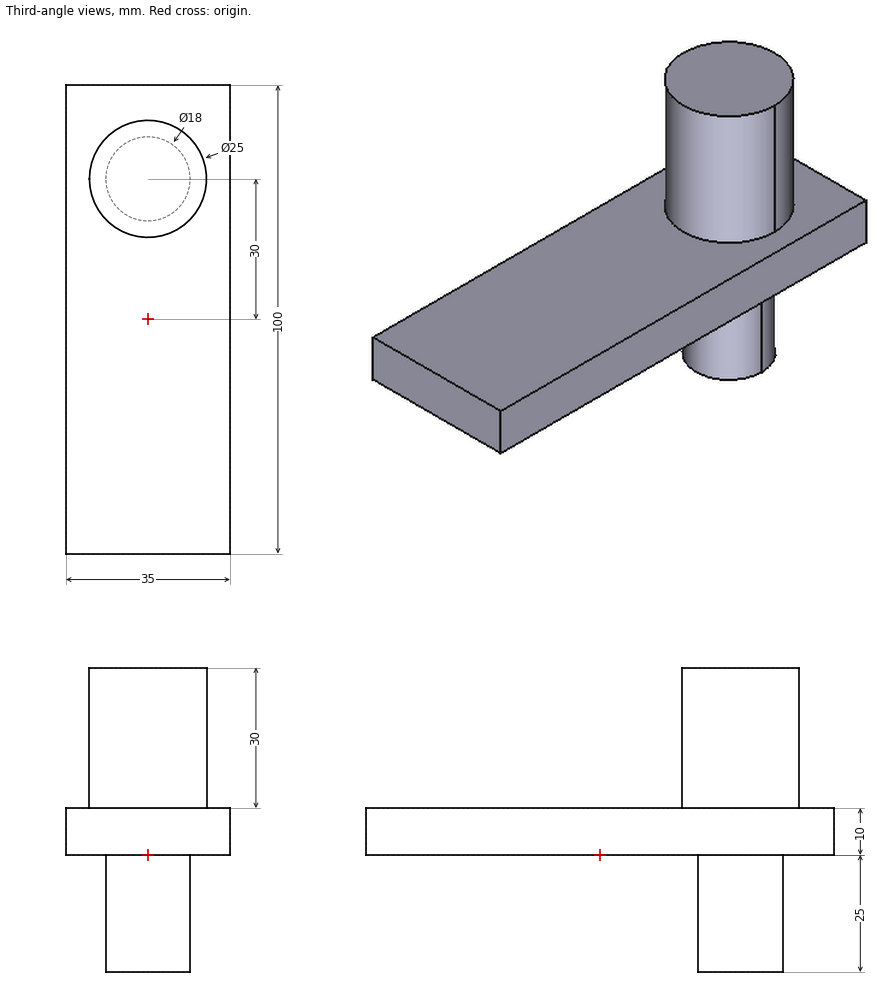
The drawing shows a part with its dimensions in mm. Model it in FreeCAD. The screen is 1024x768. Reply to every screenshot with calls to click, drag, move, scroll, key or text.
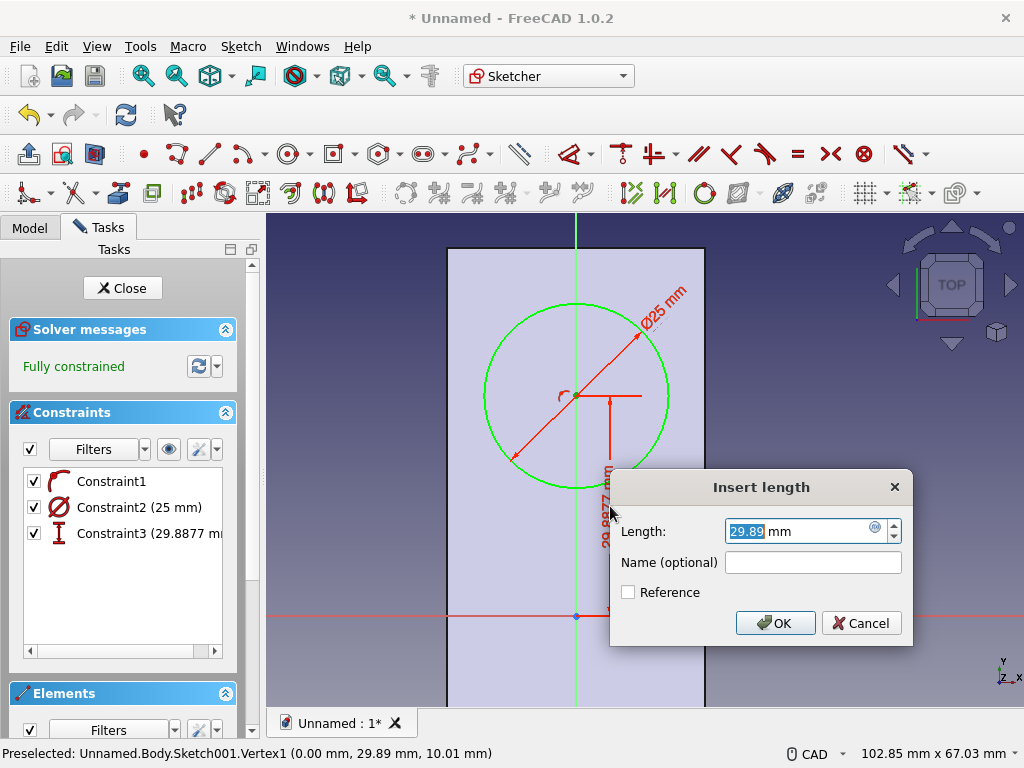
text(30)
key(Return)
key(Escape)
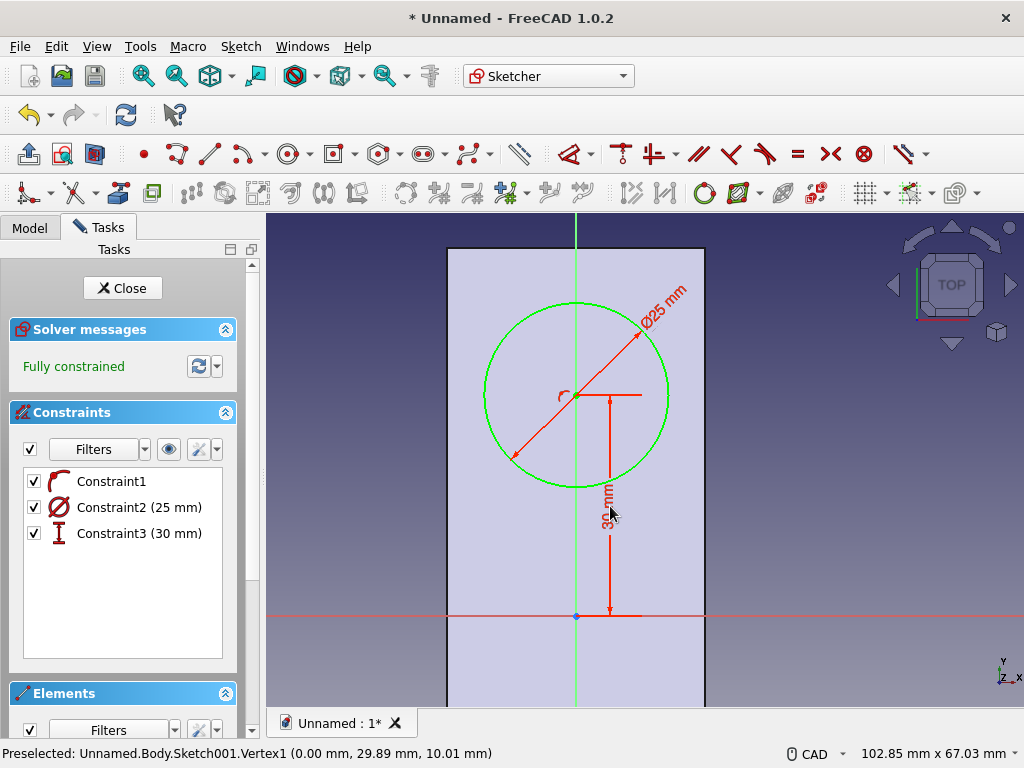
click(123, 288)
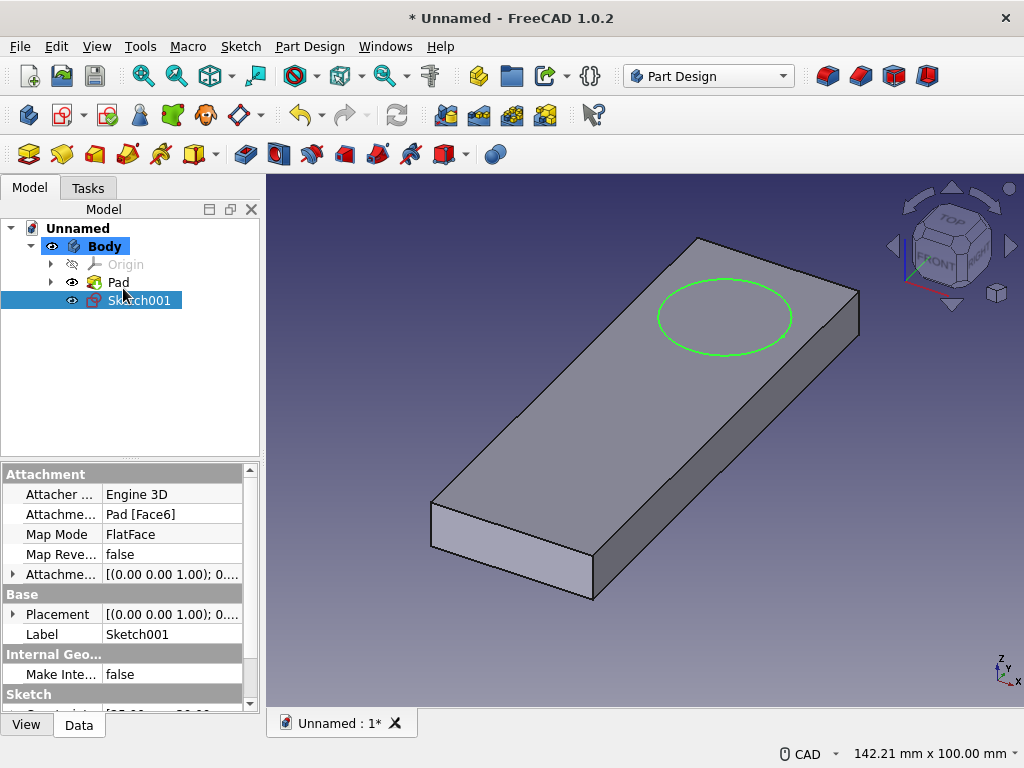
click(29, 154)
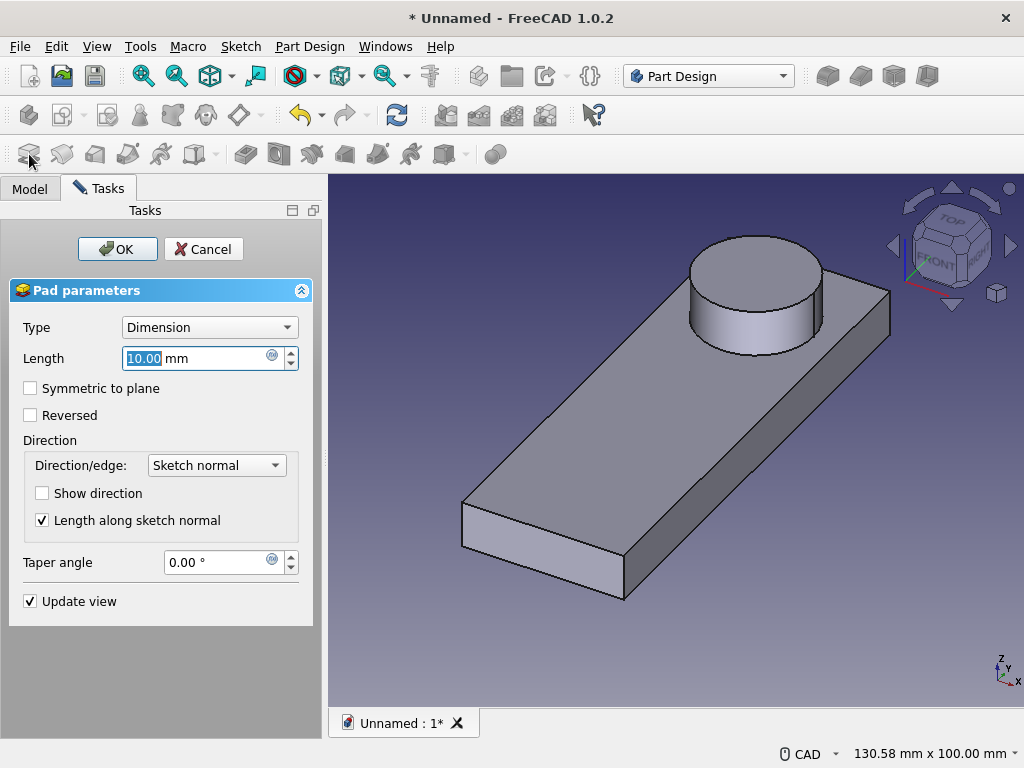
text(30)
key(Tab)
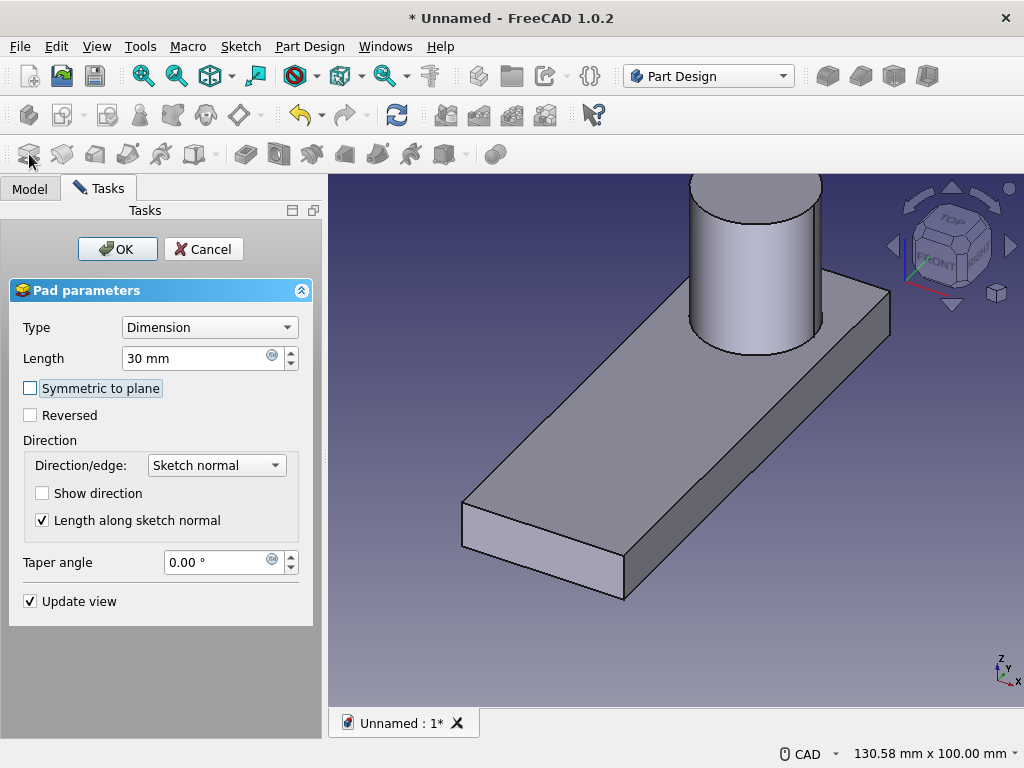
click(118, 249)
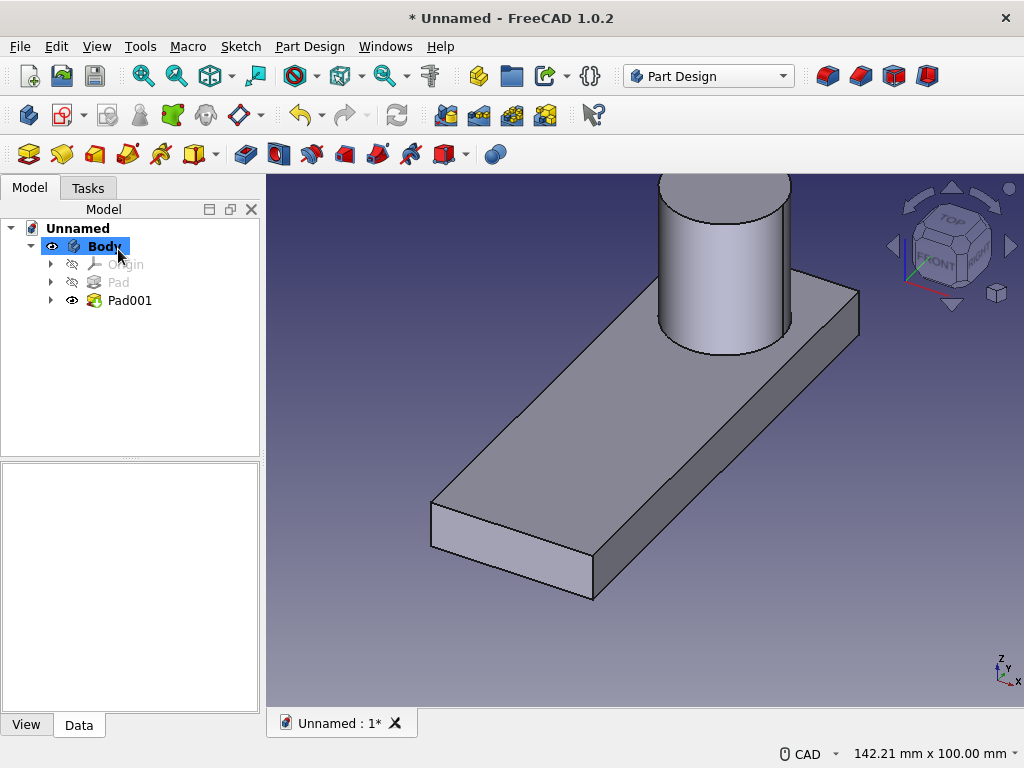
click(144, 76)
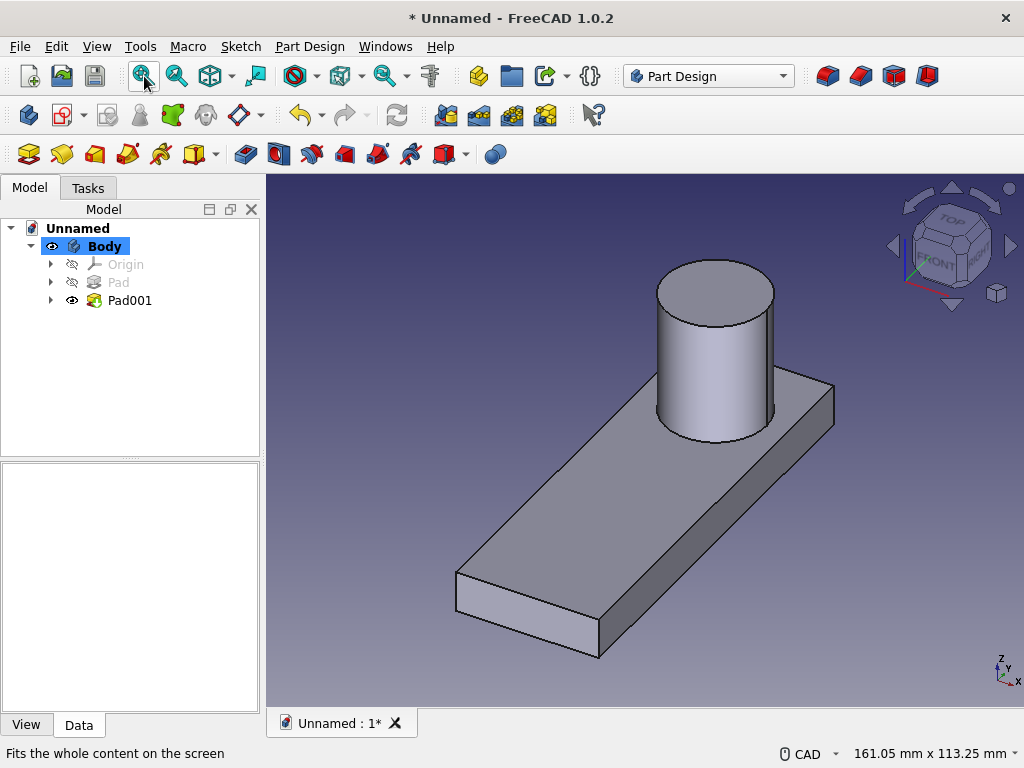
click(62, 116)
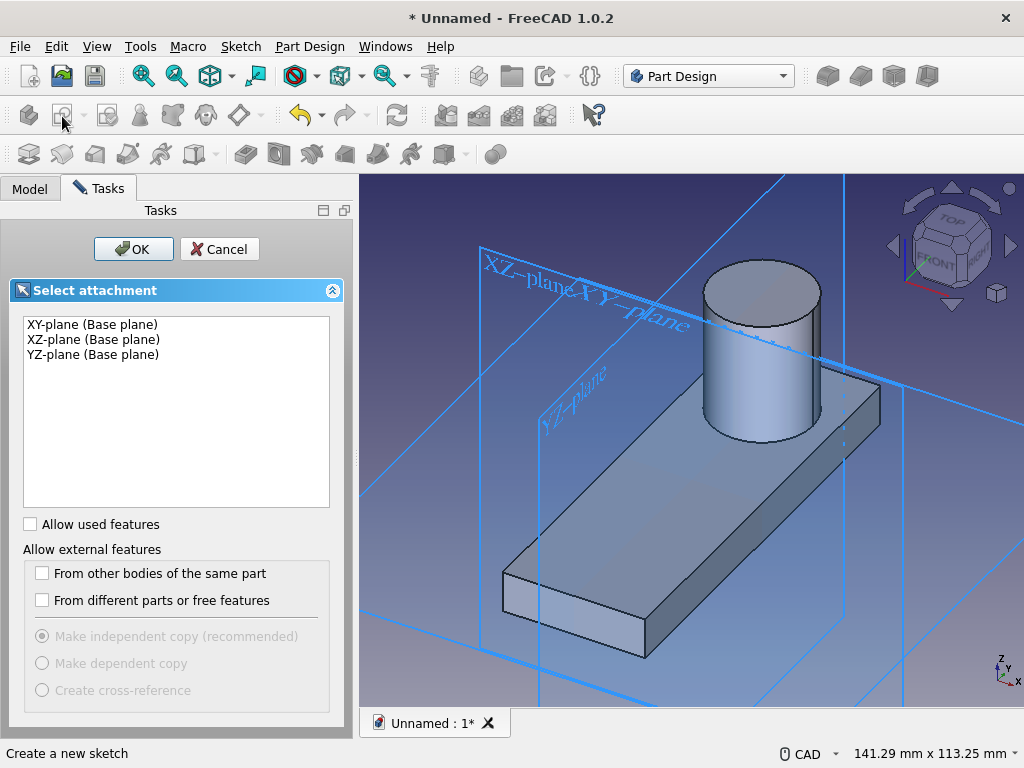
click(84, 324)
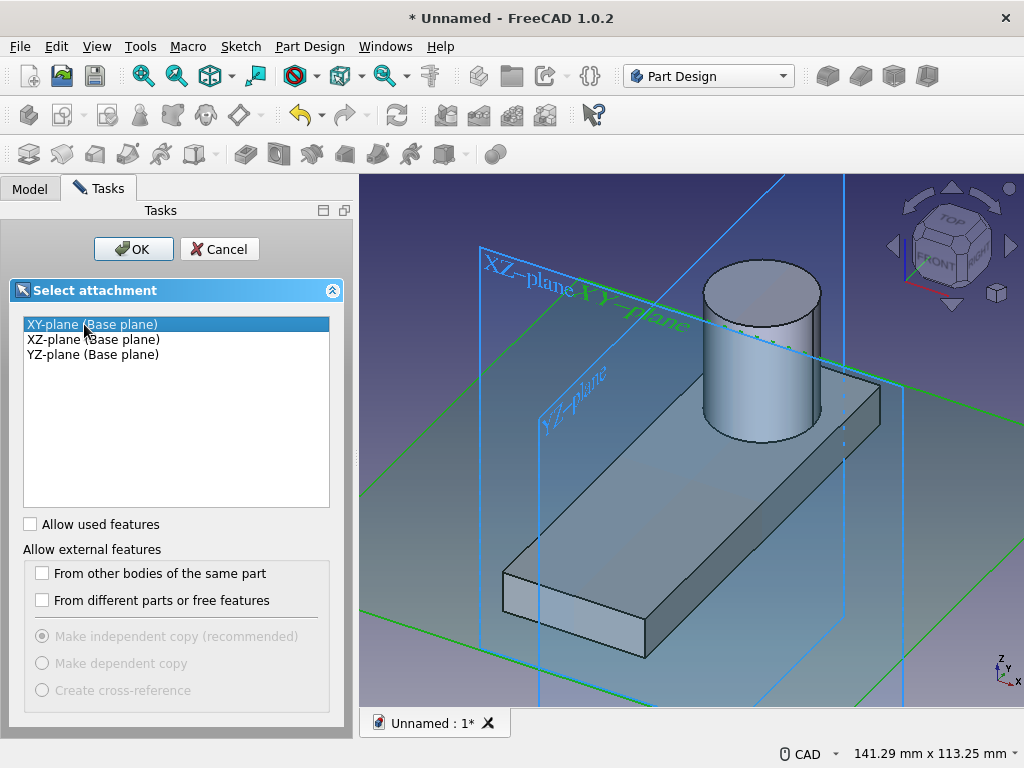
click(134, 249)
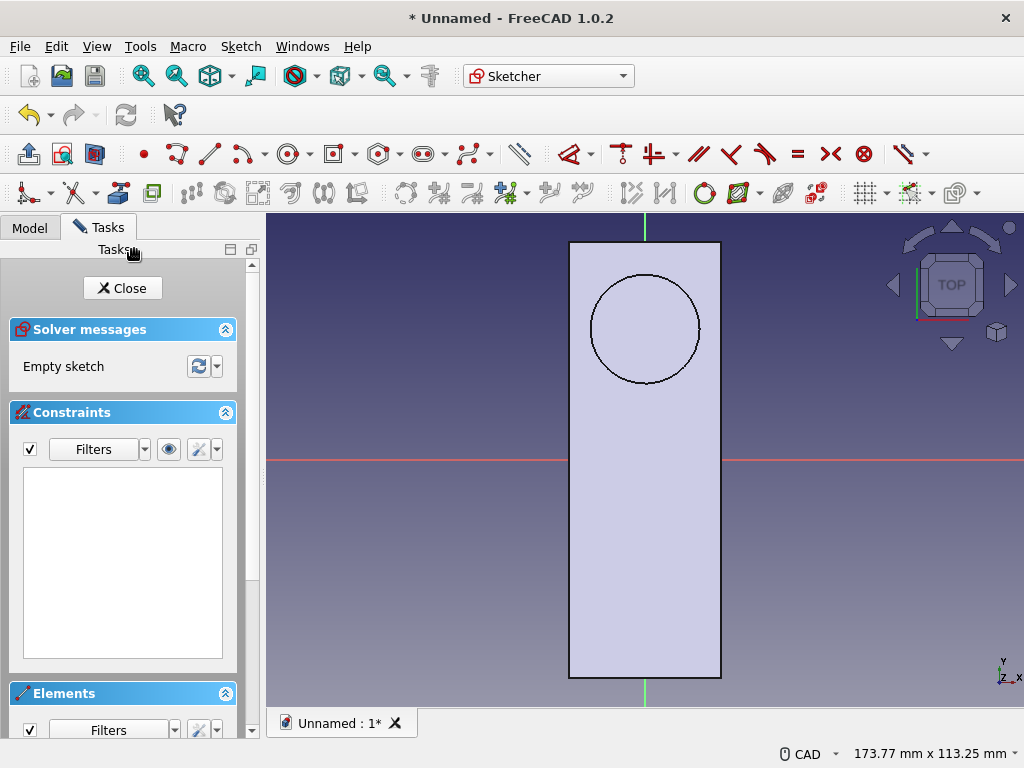
click(95, 154)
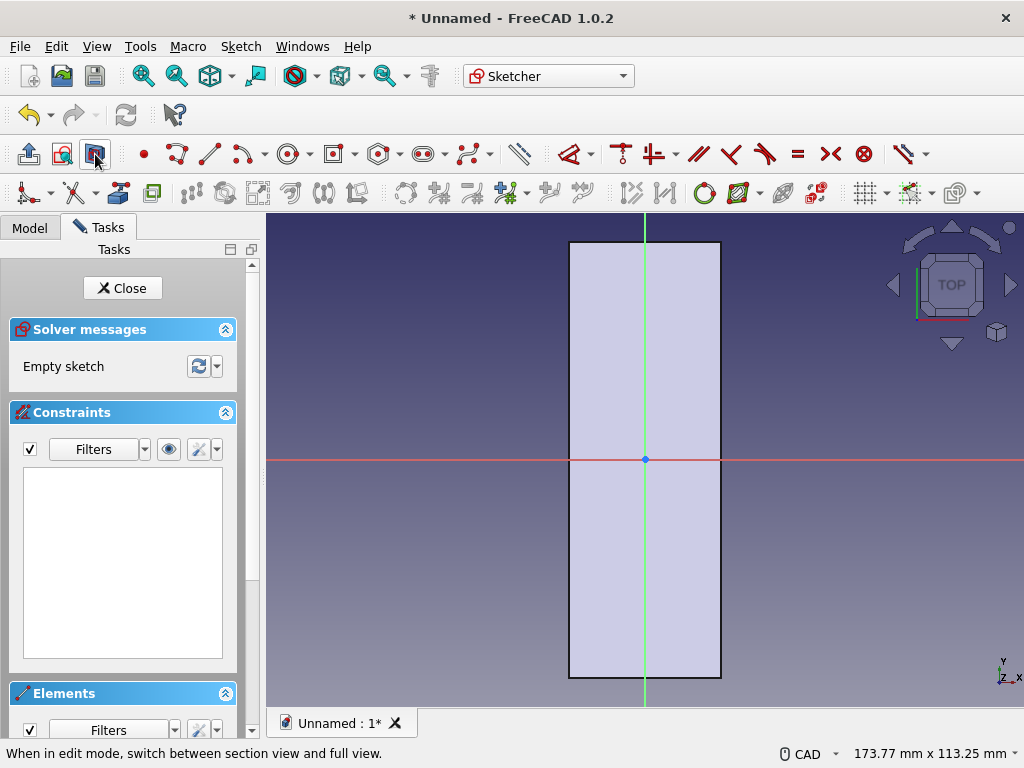
scroll(728, 271, up, 3)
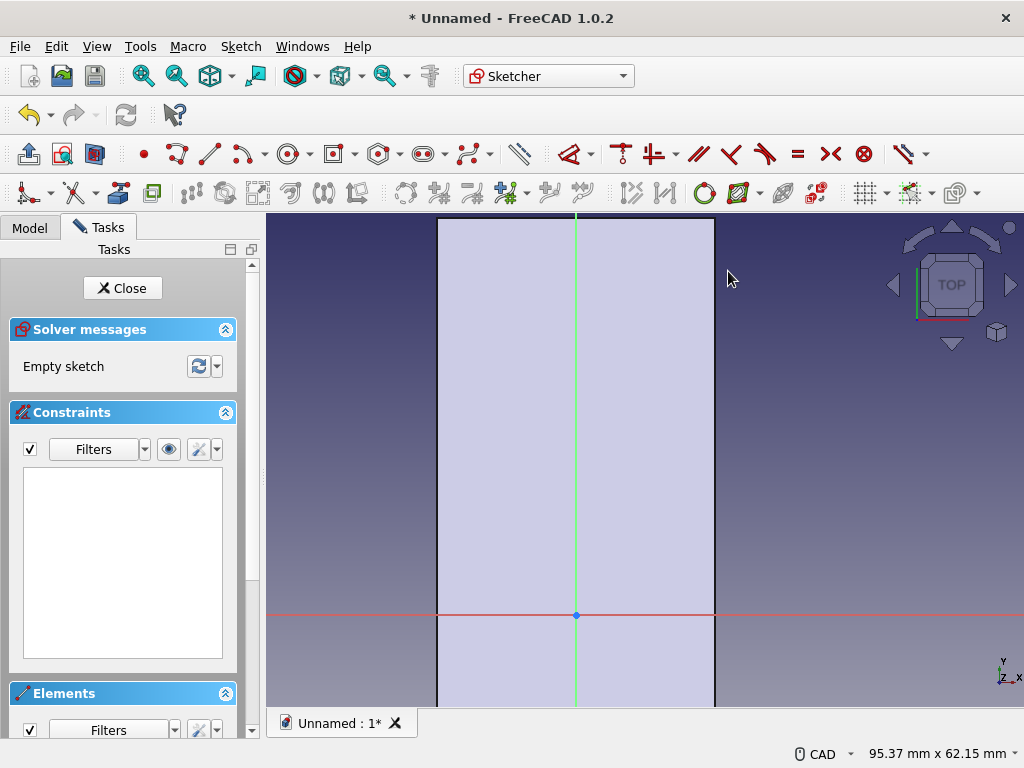
click(288, 154)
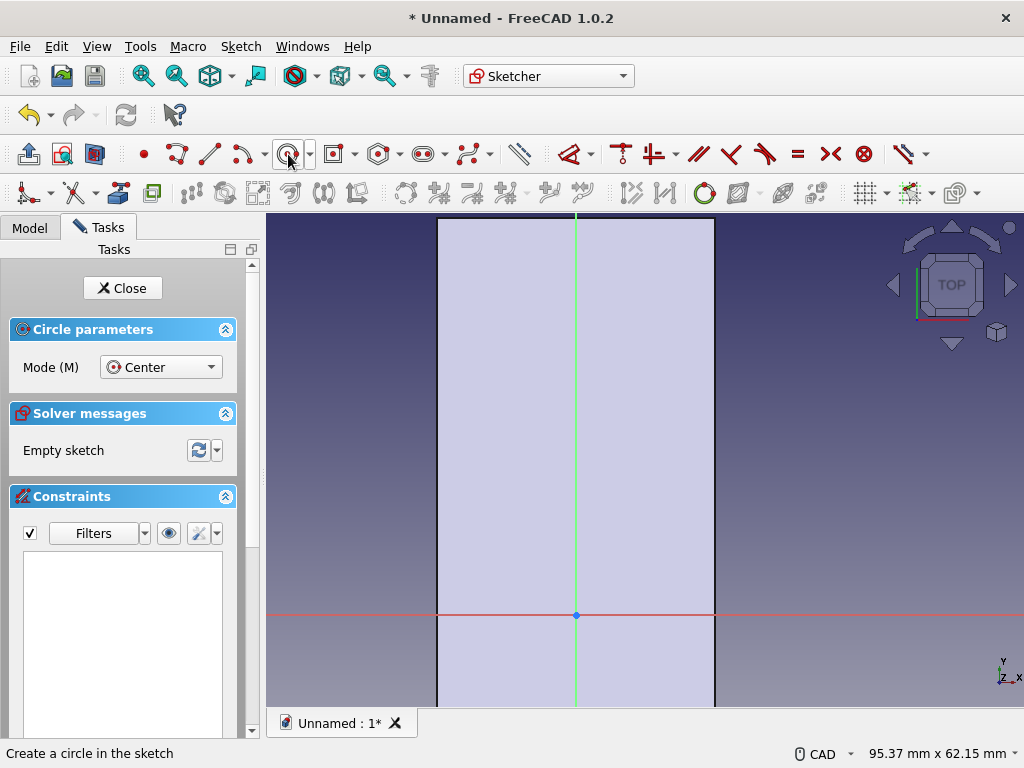
click(576, 377)
click(627, 326)
key(Escape)